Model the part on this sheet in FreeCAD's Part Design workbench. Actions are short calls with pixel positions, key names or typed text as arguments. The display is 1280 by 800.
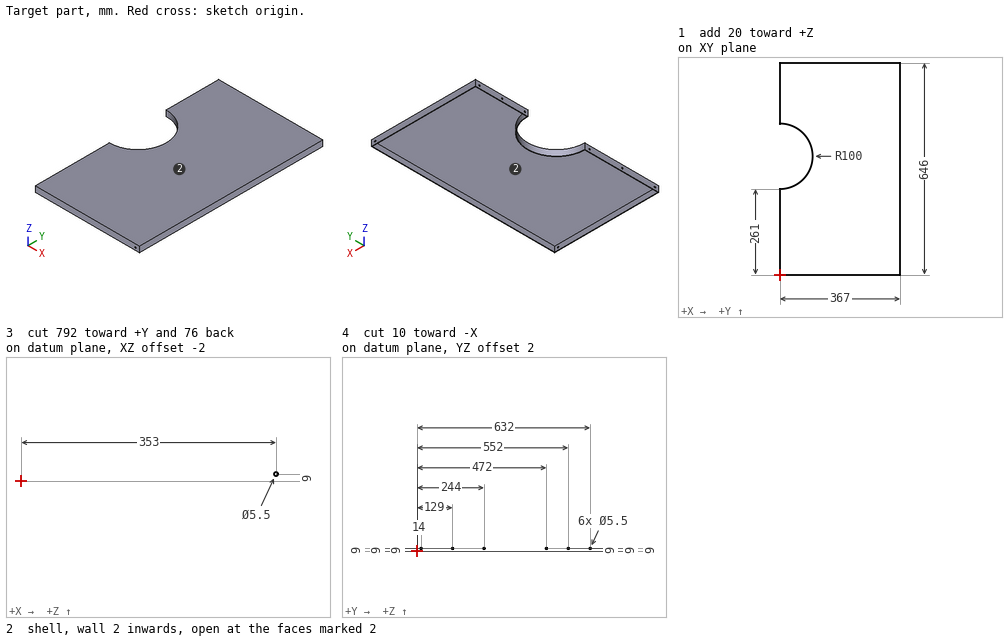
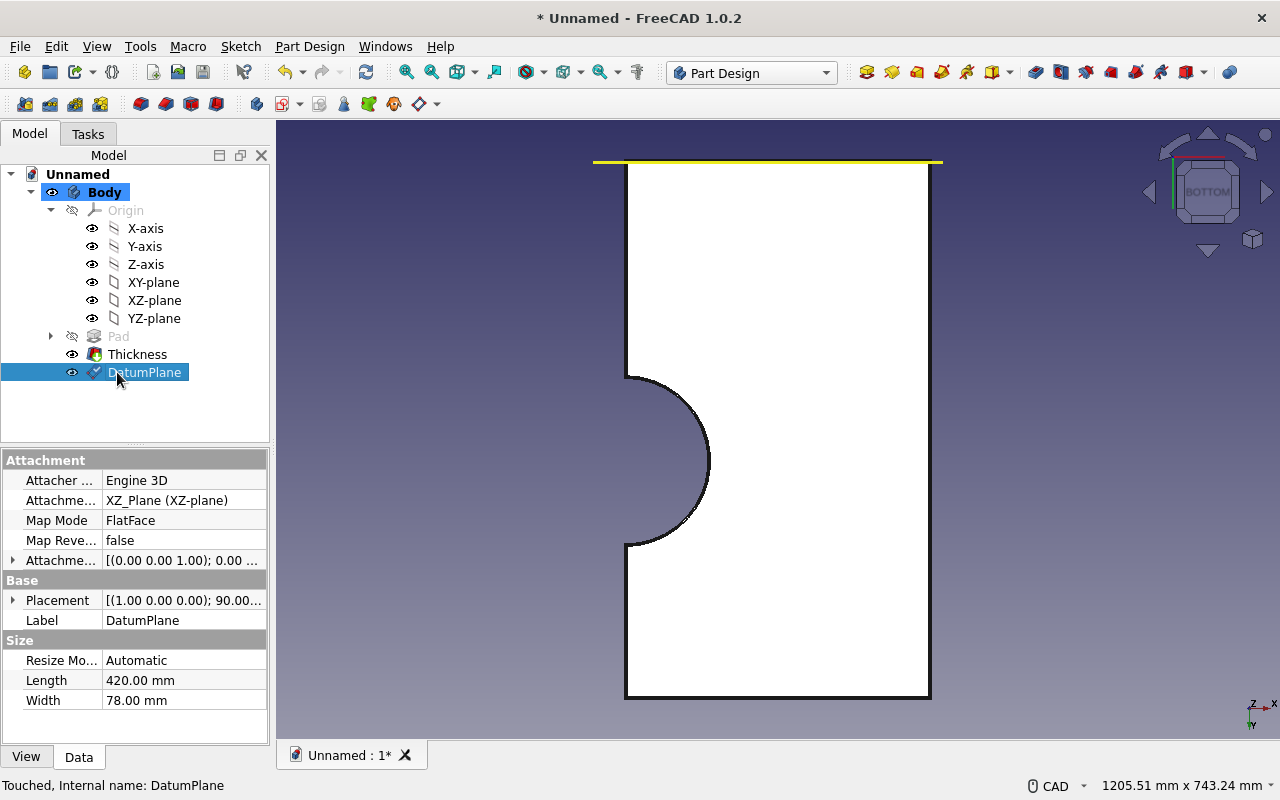
click(282, 104)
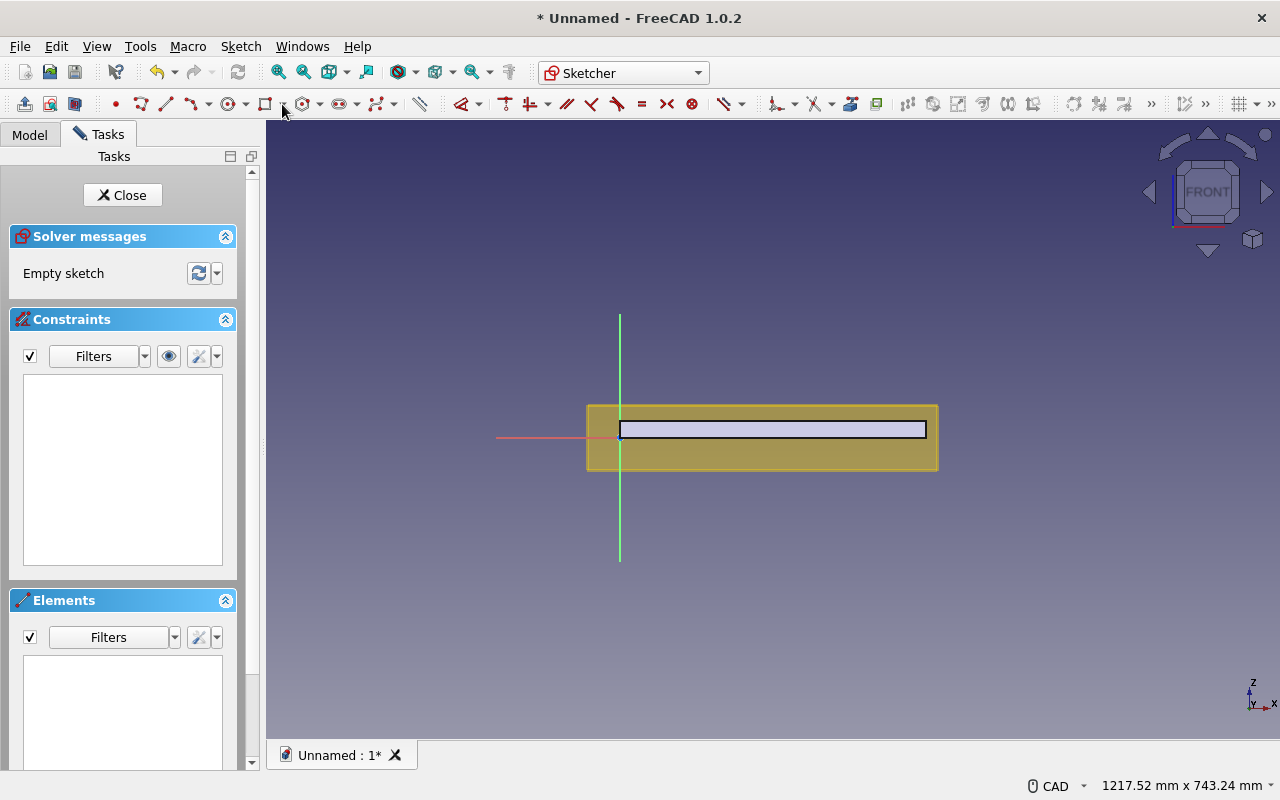
click(75, 104)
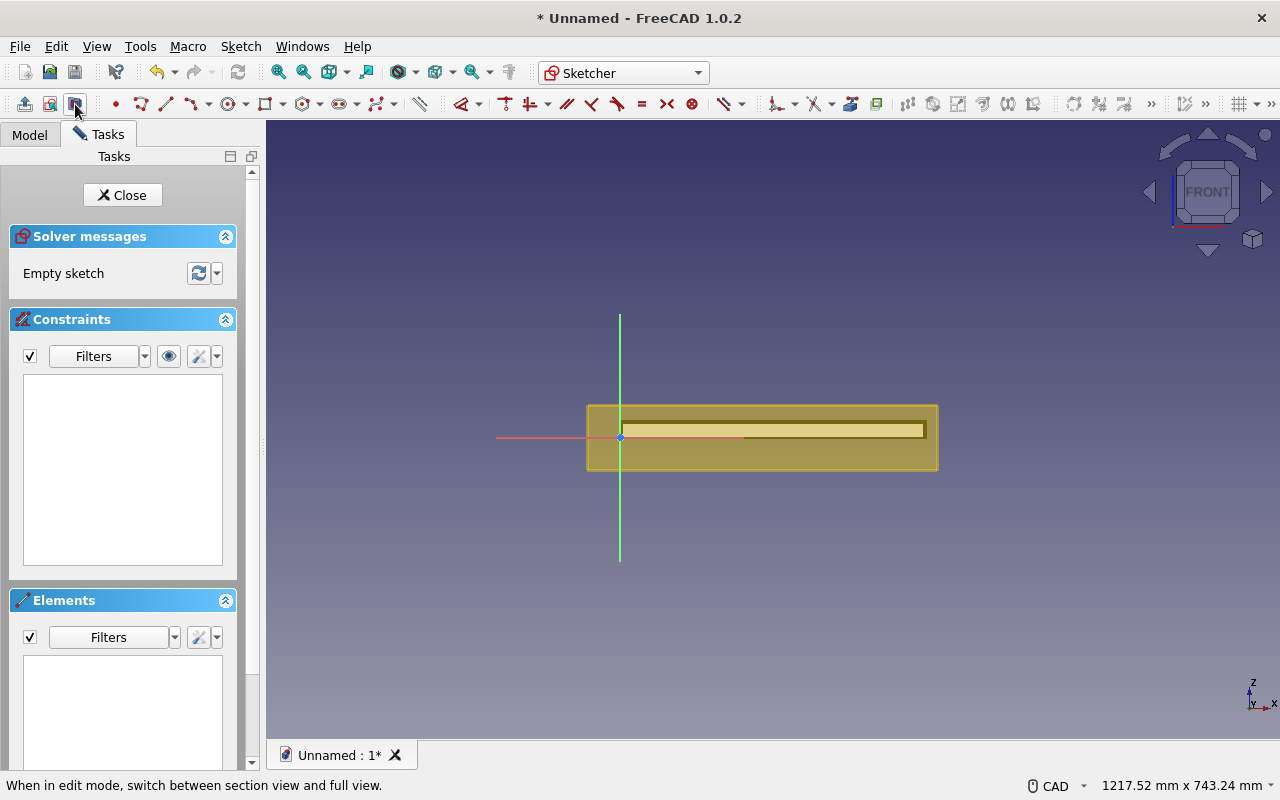
scroll(925, 430, up, 15)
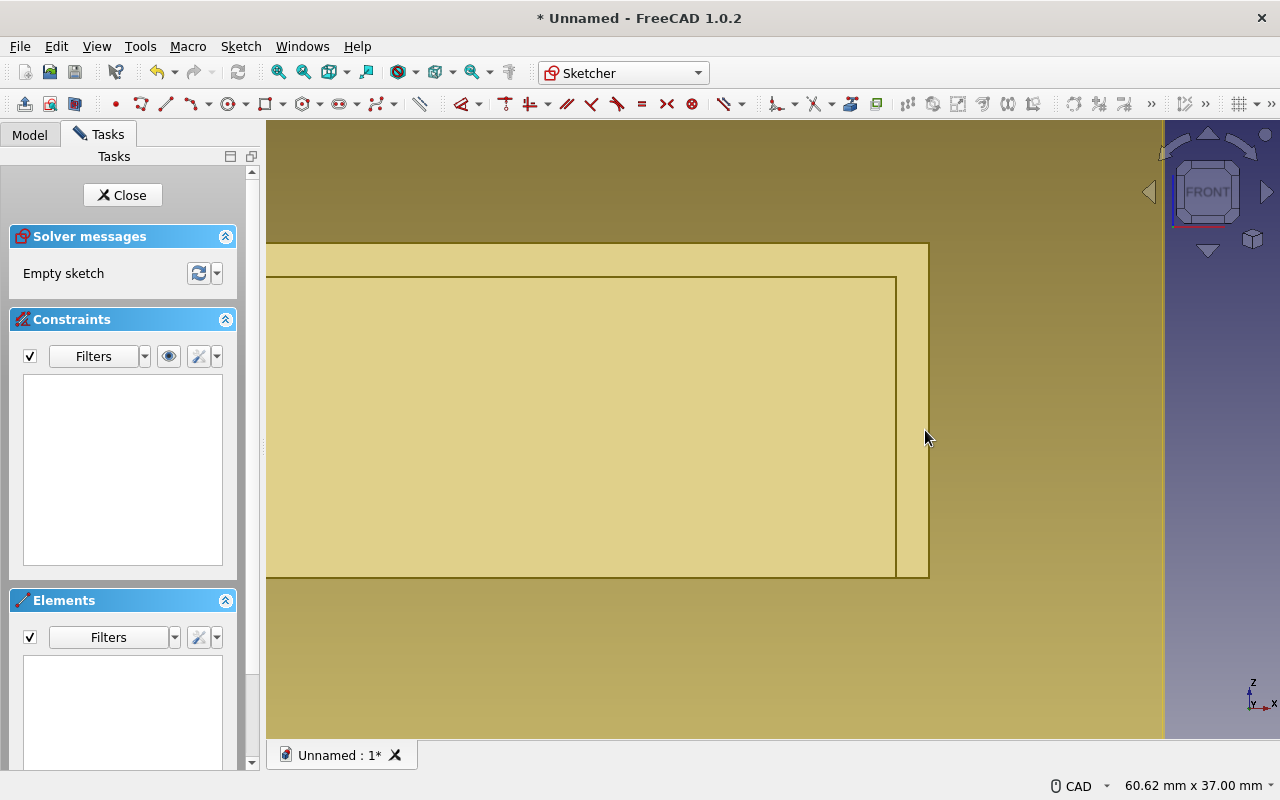
scroll(692, 426, up, 7)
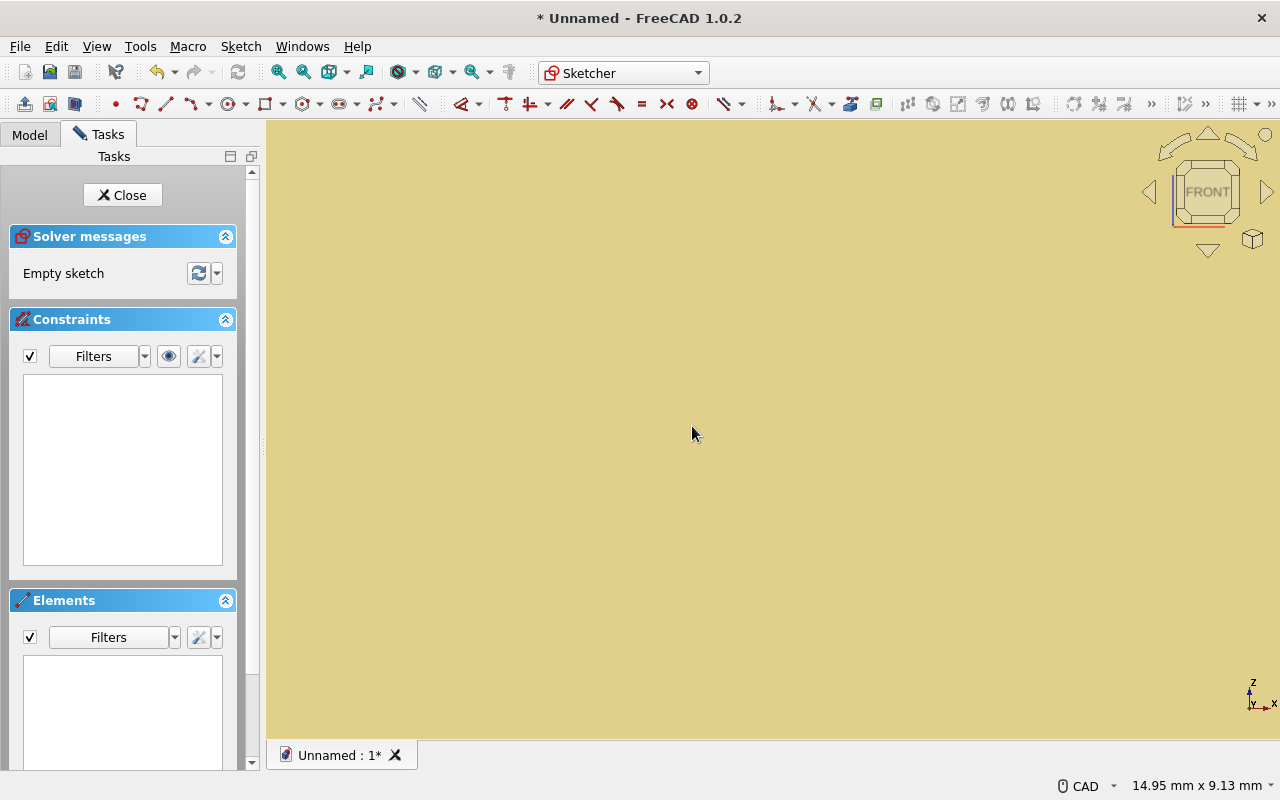
click(228, 104)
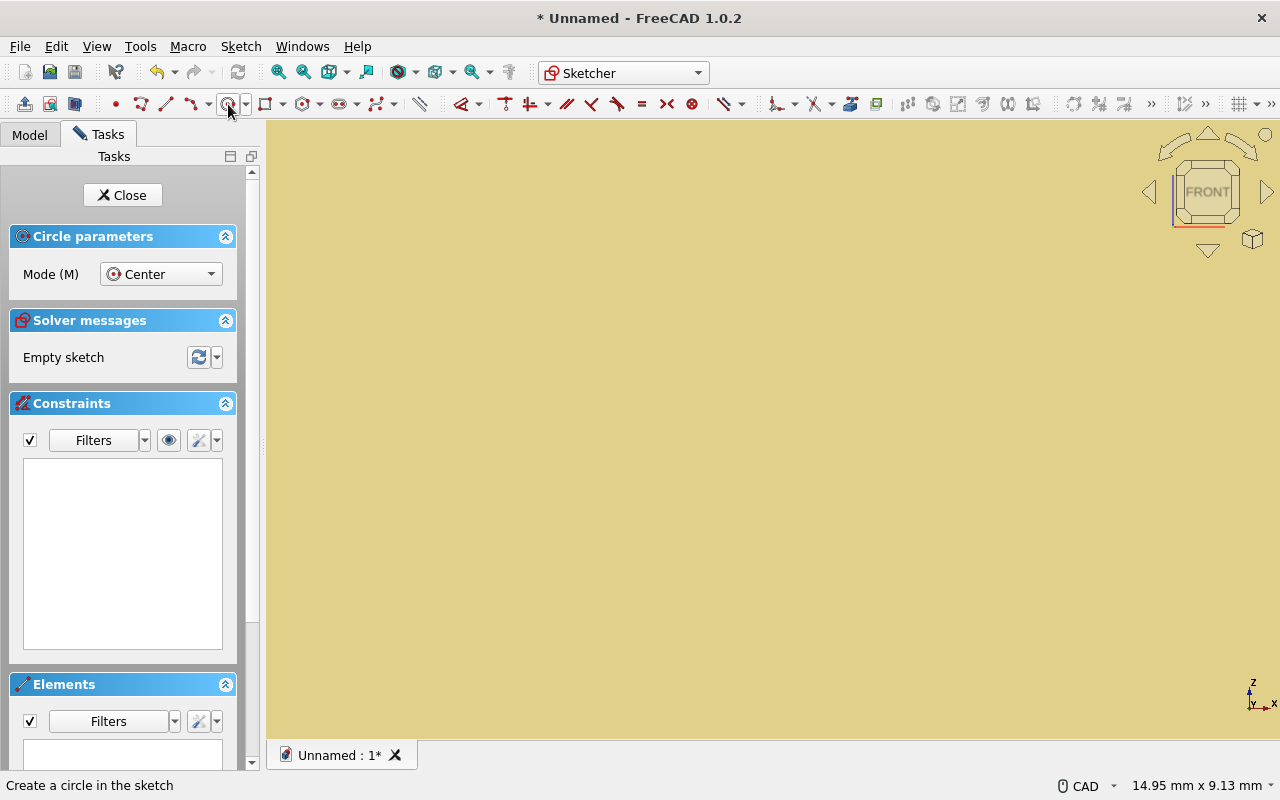
click(703, 429)
click(835, 297)
key(Escape)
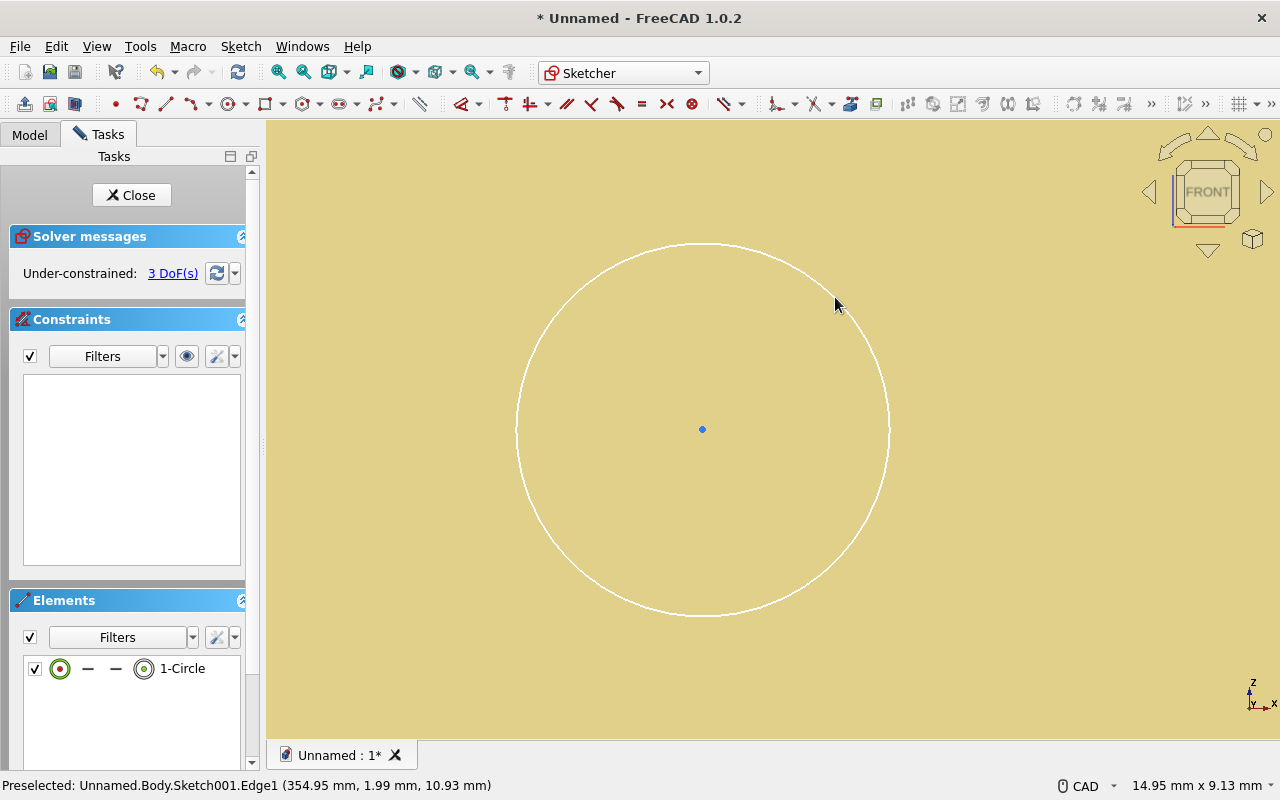
click(460, 104)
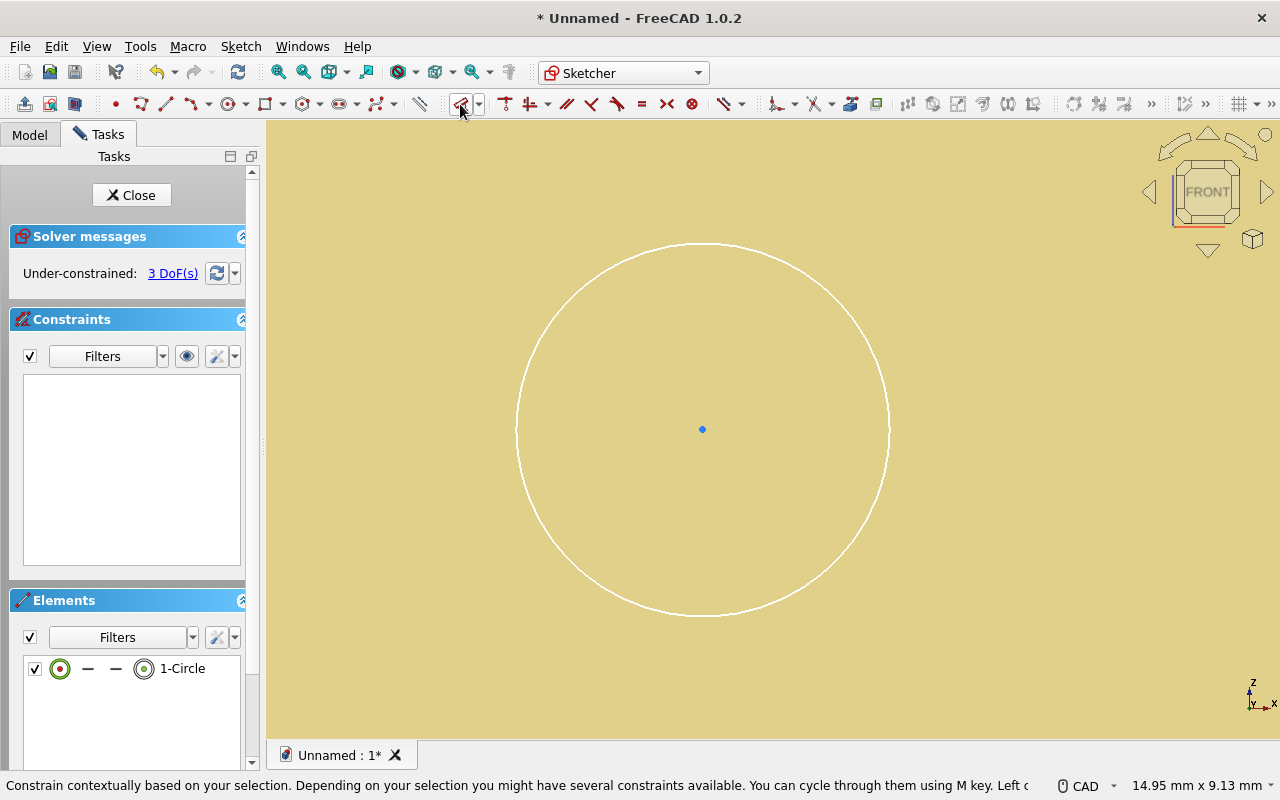
click(835, 298)
click(858, 275)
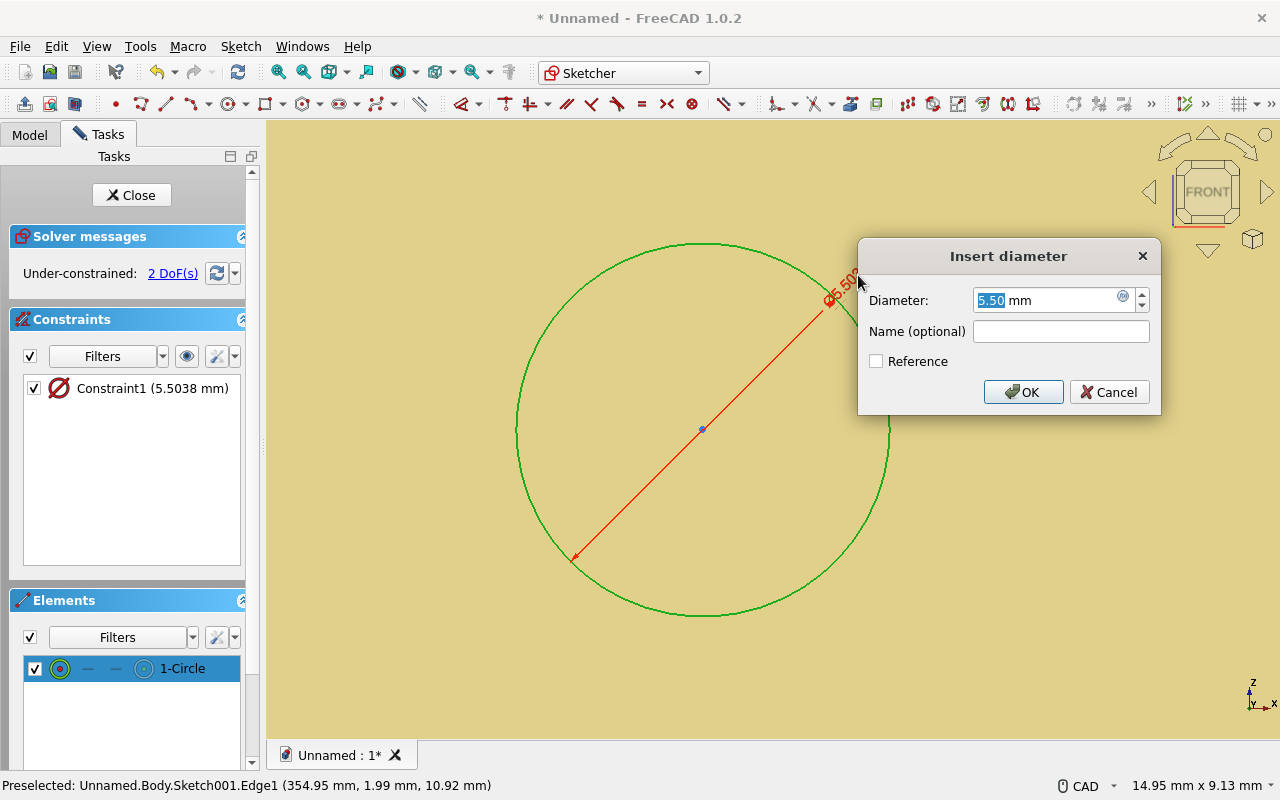
text(5.5)
key(Return)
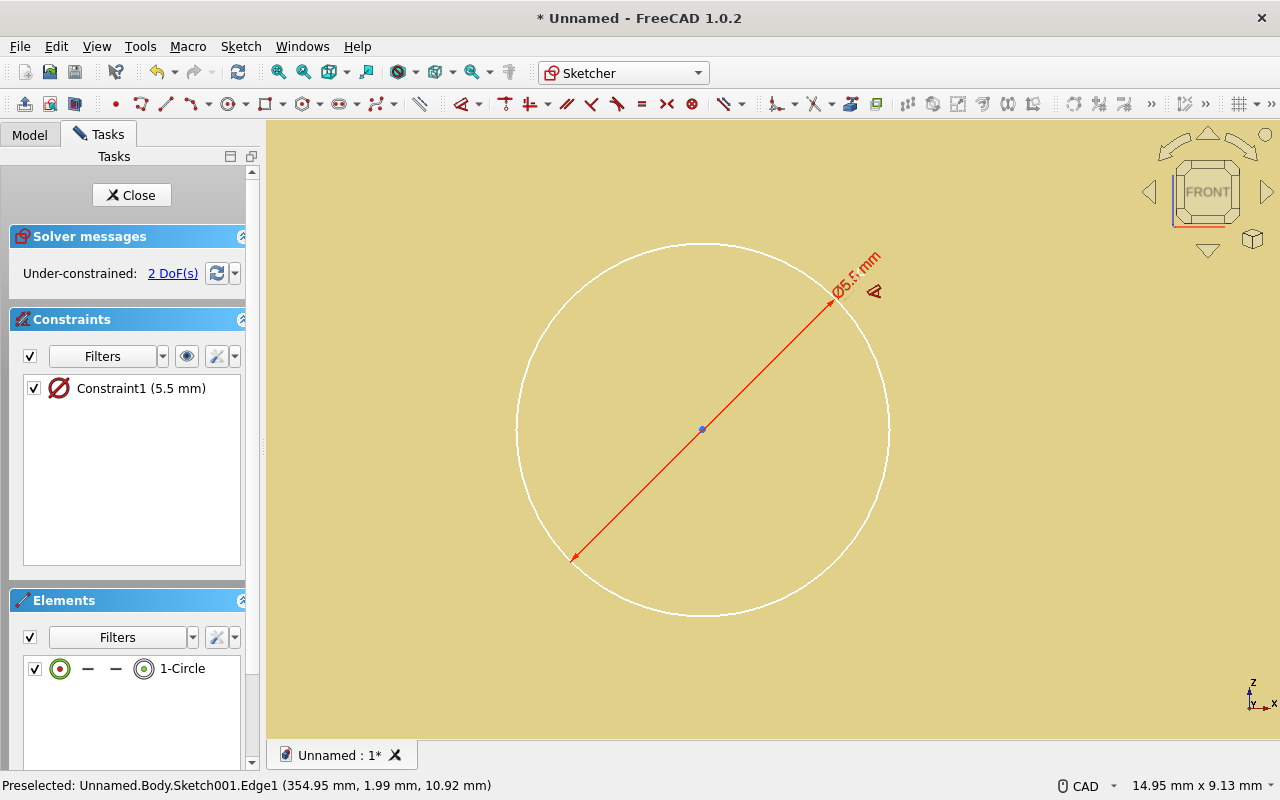
click(703, 430)
click(737, 571)